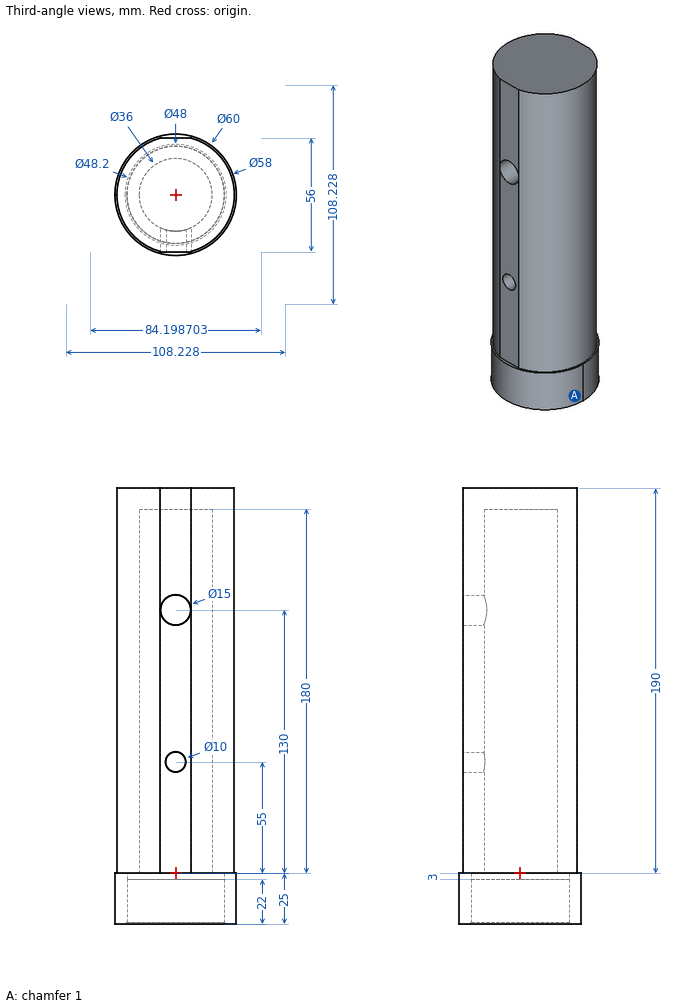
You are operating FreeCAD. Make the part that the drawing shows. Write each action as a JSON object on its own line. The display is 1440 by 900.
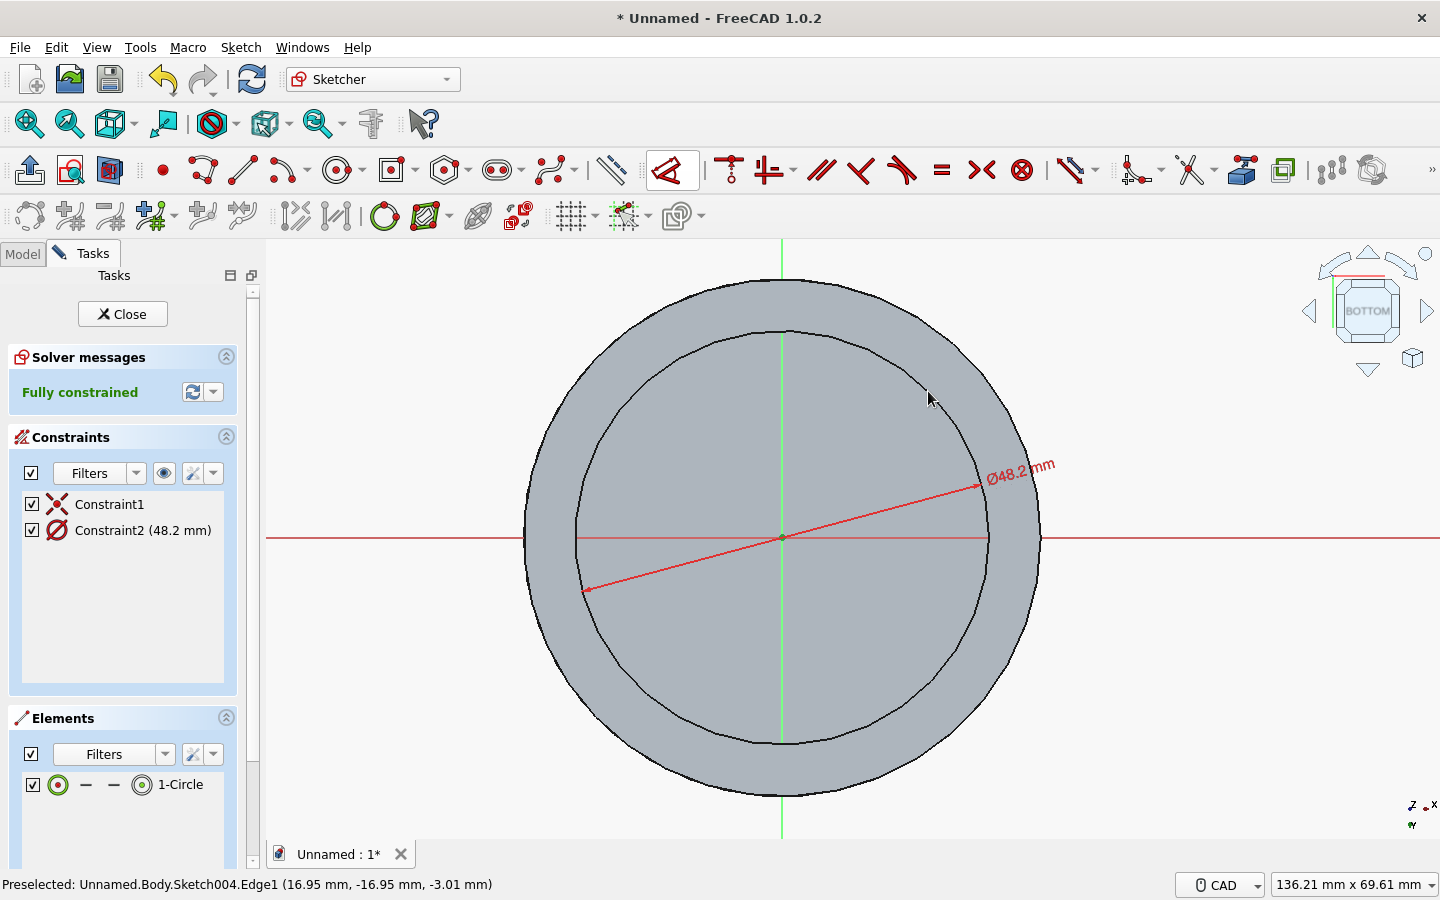
{"action": "left_click", "coordinate": [123, 314]}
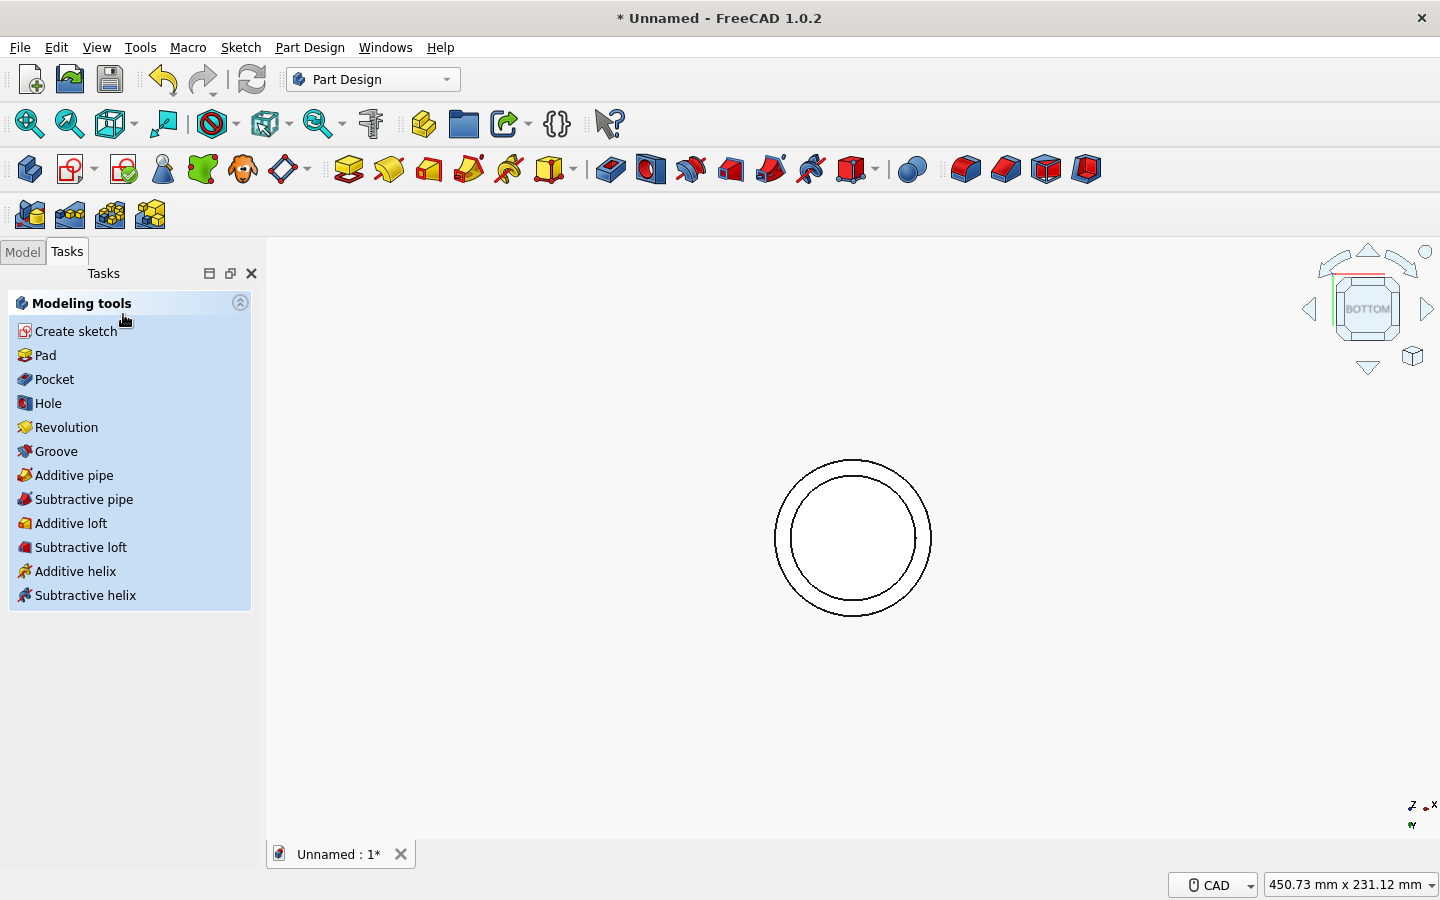
{"action": "left_click", "coordinate": [612, 170]}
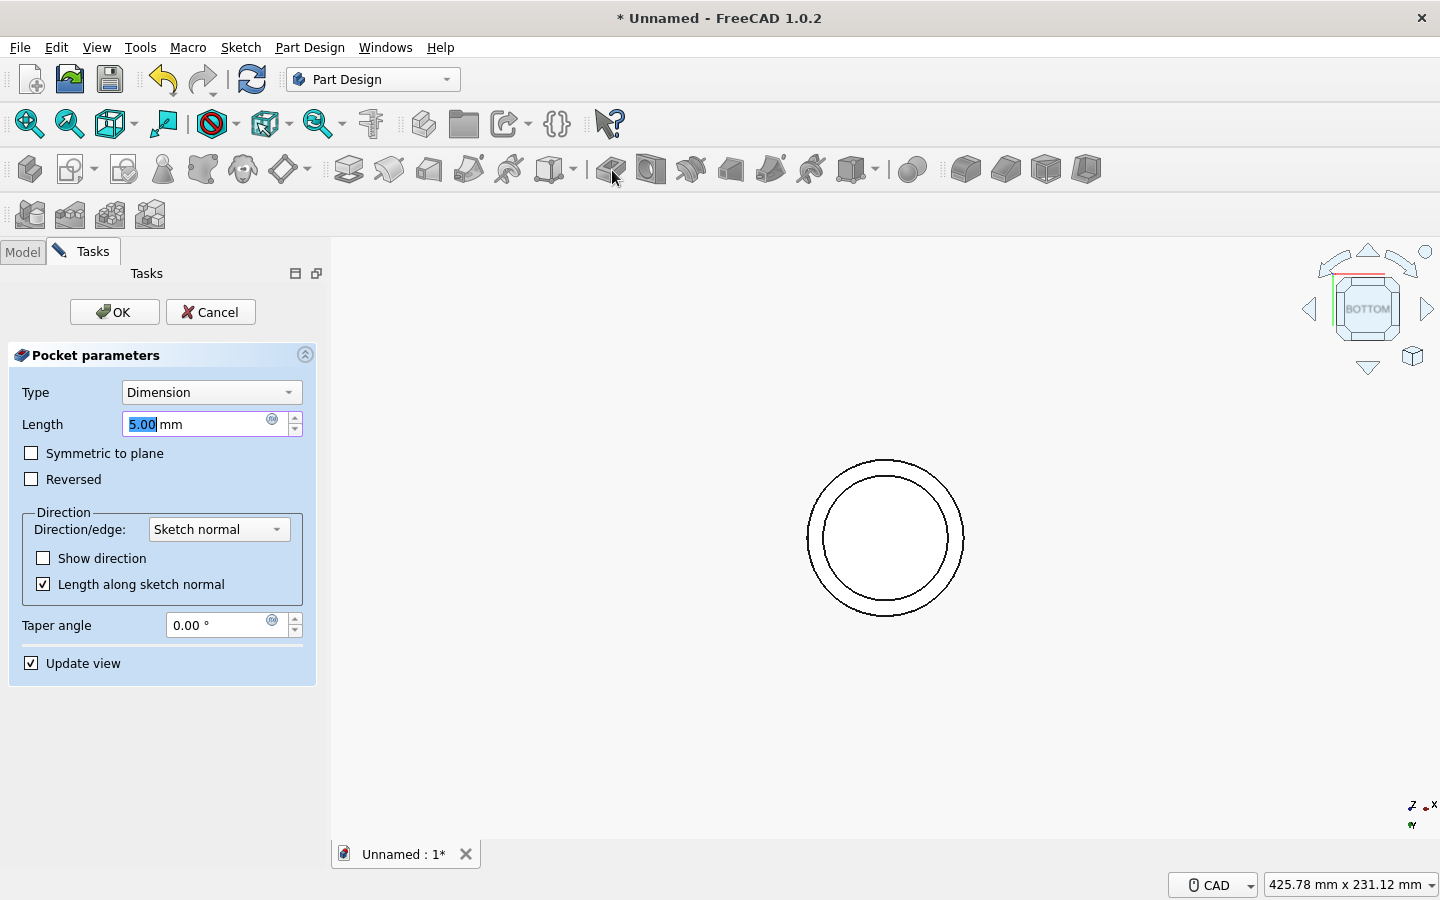
{"action": "type", "text": "3"}
{"action": "key", "text": "Tab"}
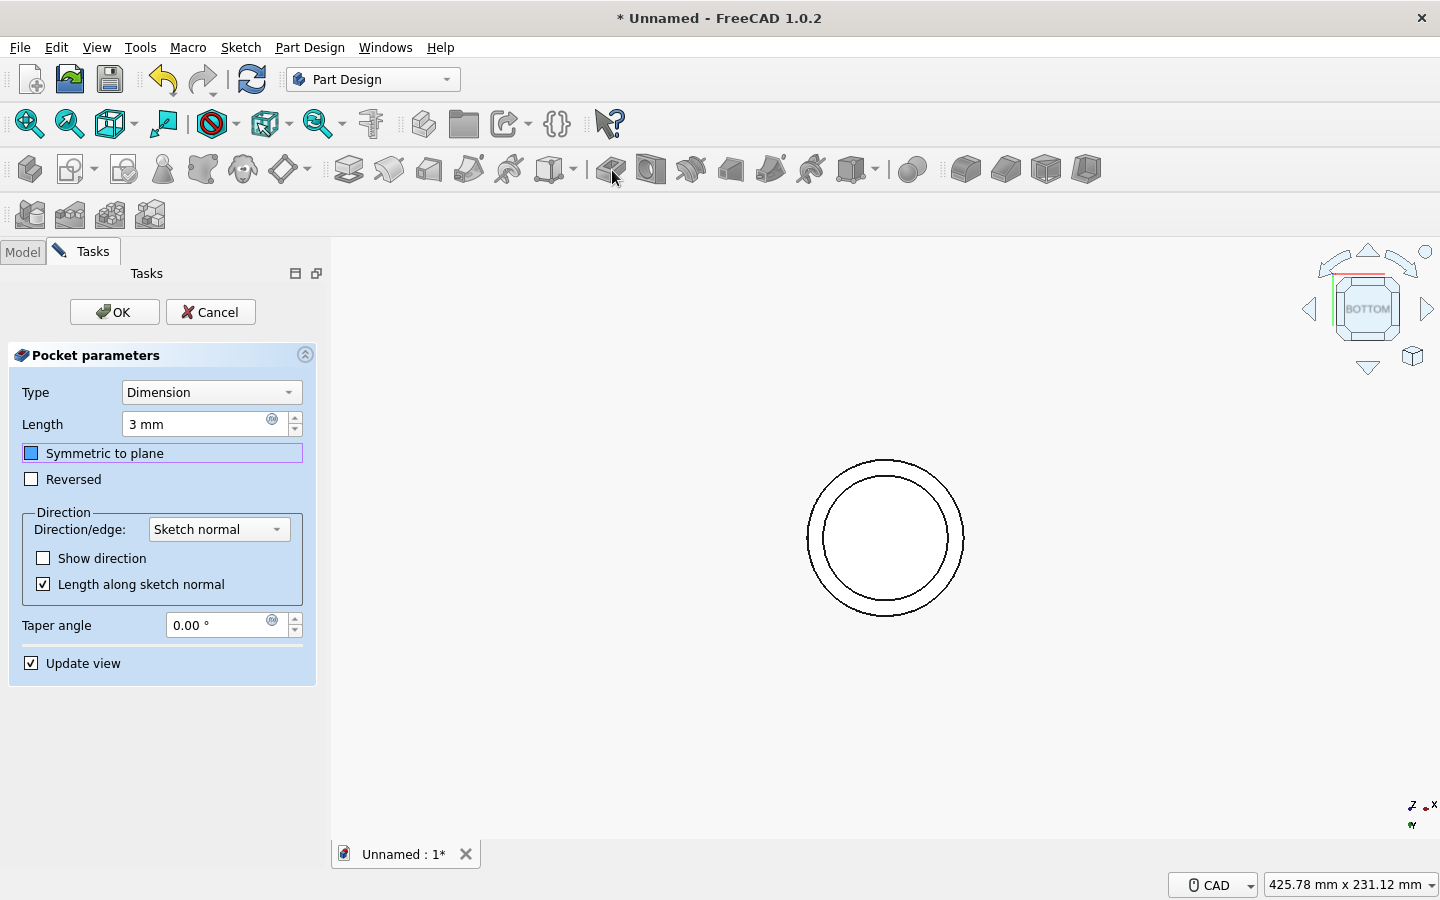
{"action": "left_click", "coordinate": [115, 312]}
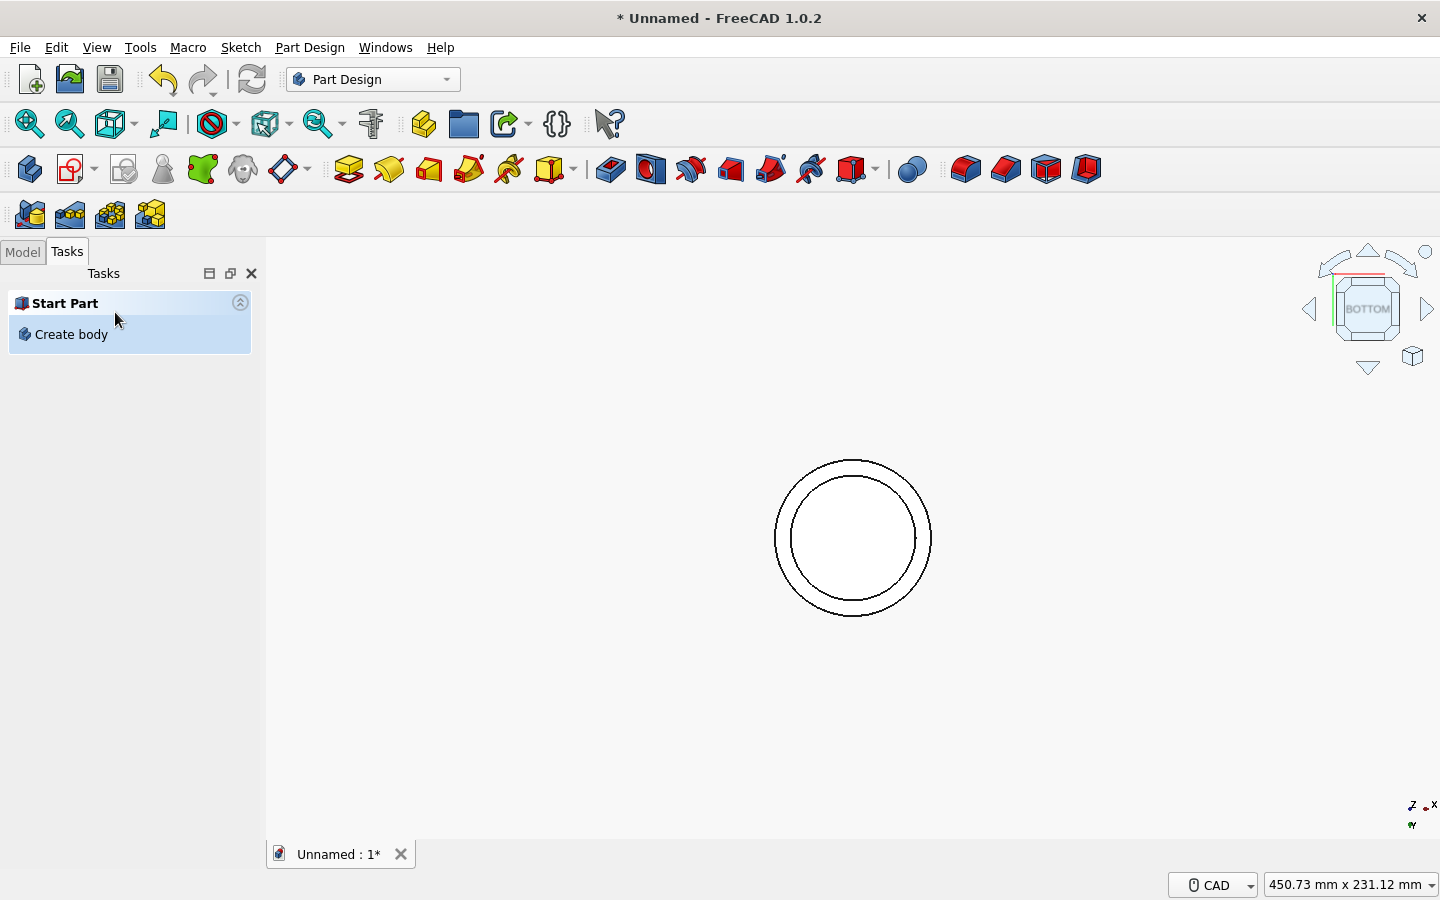
{"action": "left_click", "coordinate": [30, 124]}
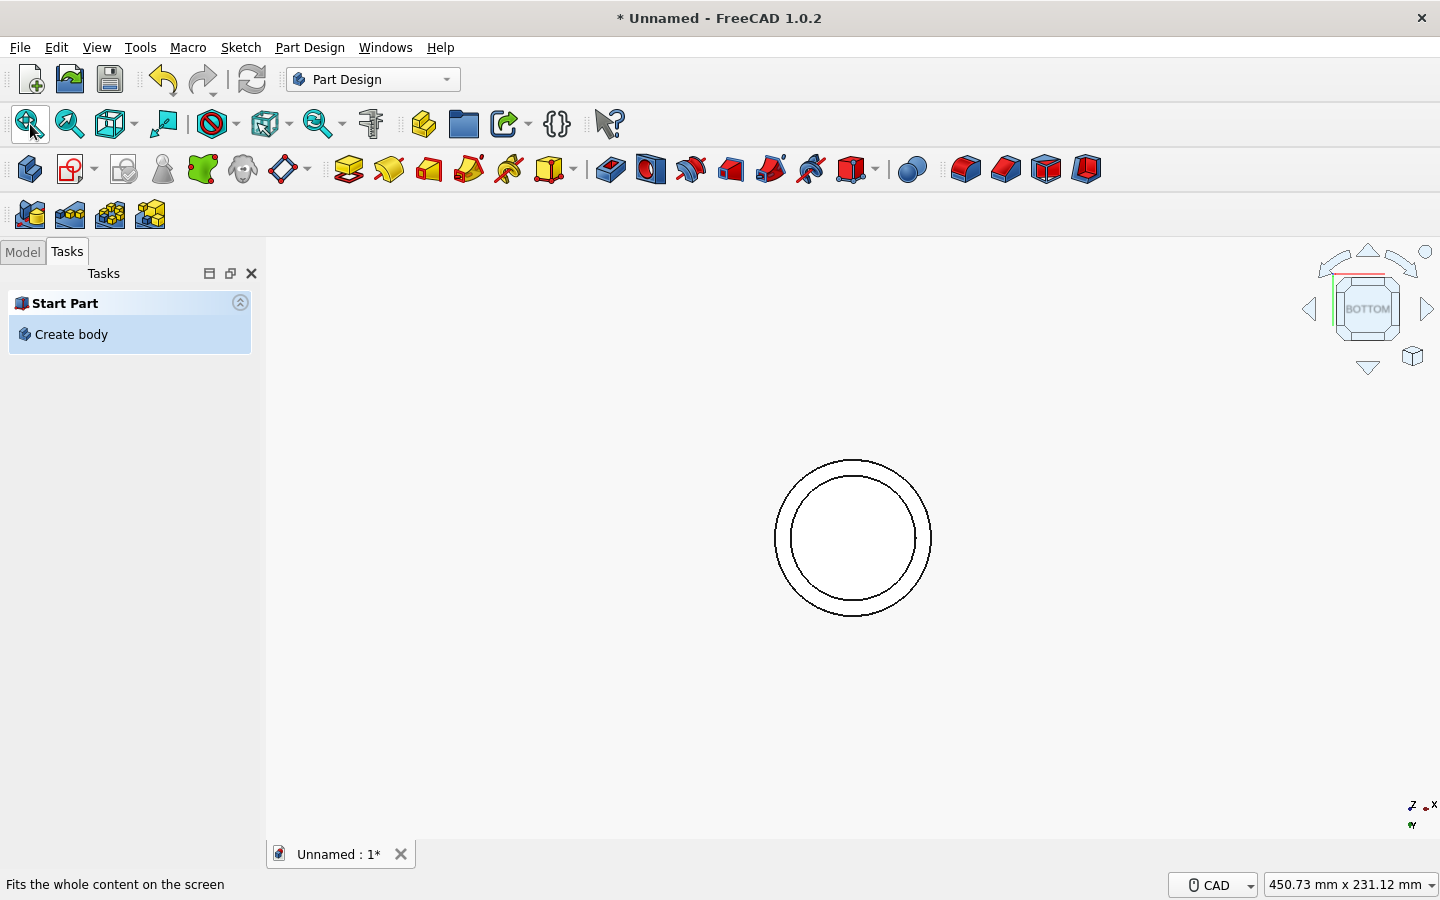
{"action": "left_click", "coordinate": [70, 170]}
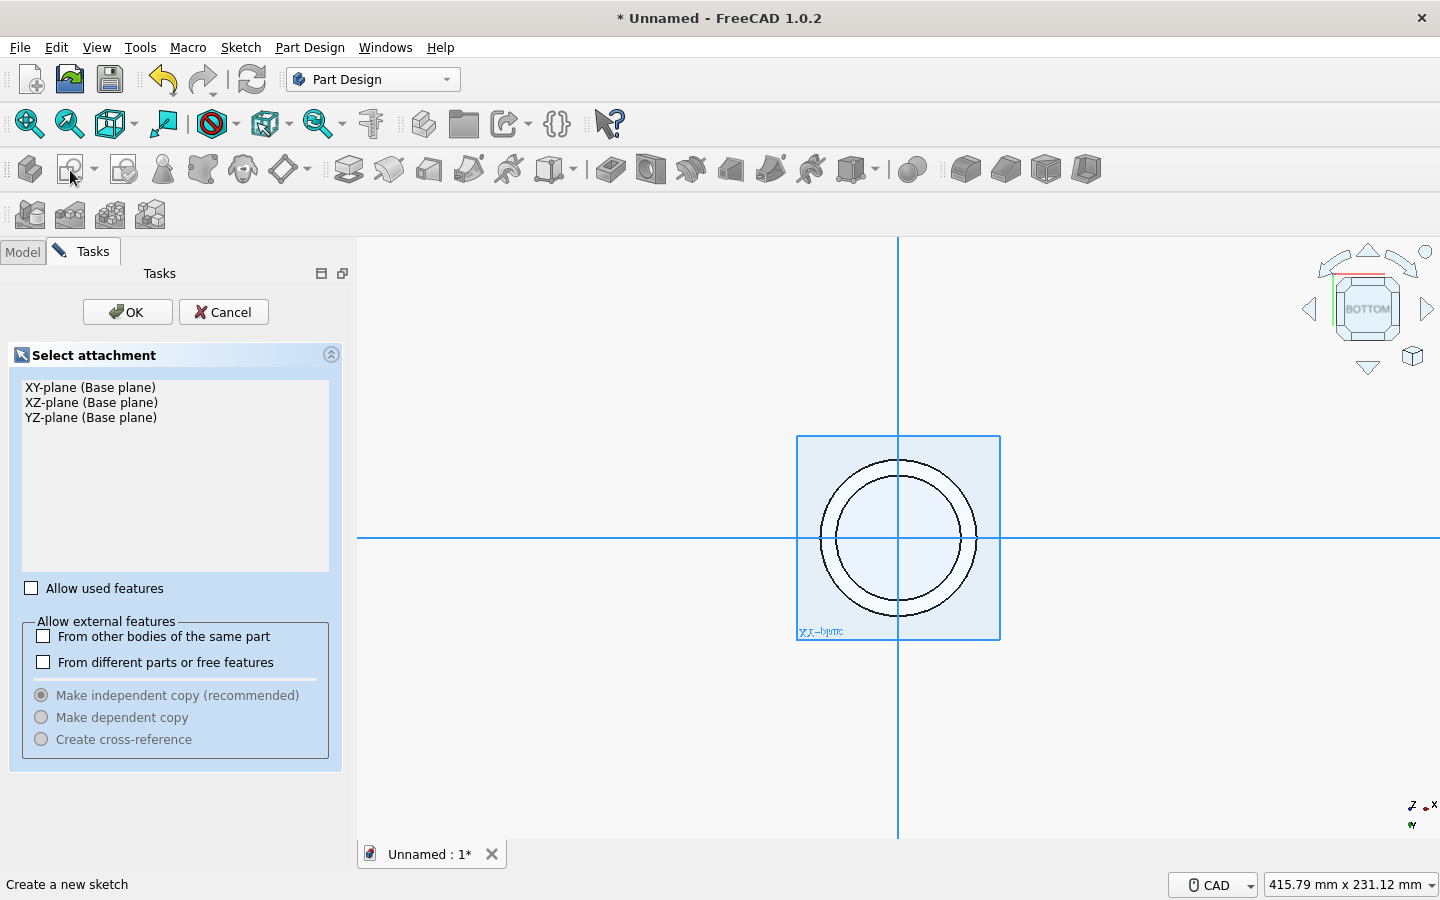
{"action": "left_click", "coordinate": [82, 388]}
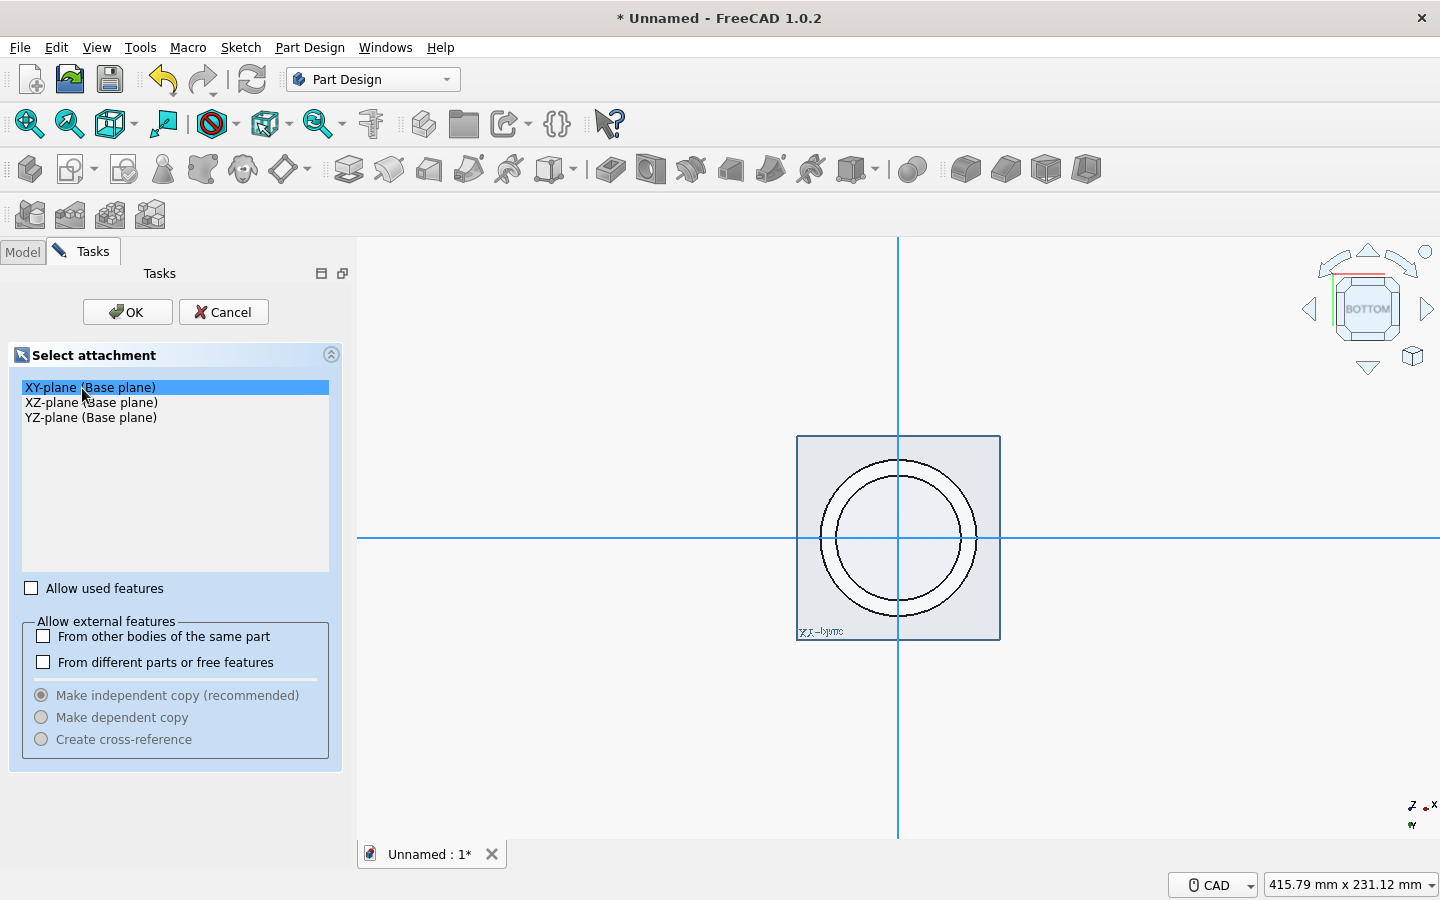
{"action": "left_click", "coordinate": [128, 312]}